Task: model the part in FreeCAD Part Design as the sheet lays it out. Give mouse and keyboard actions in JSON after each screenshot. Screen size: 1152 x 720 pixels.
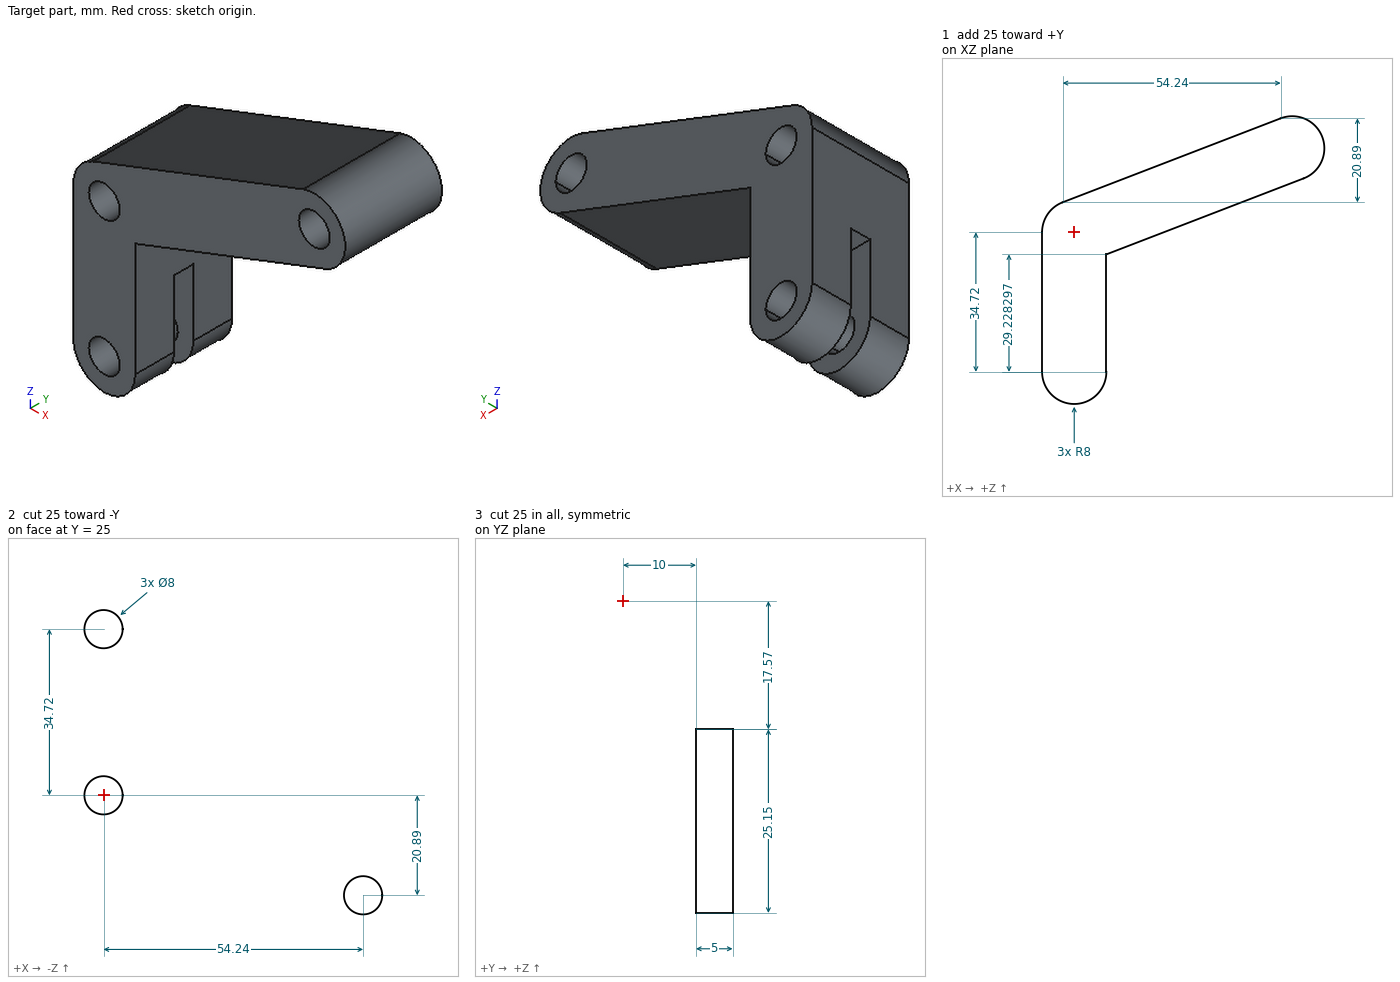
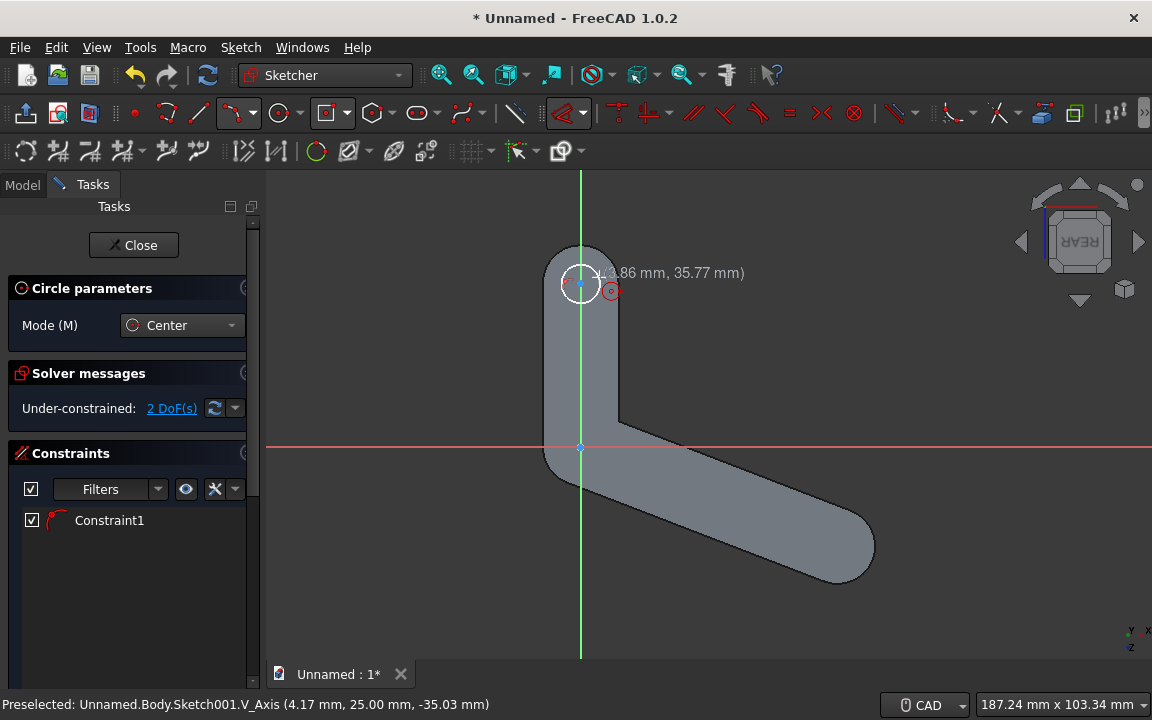
{"action": "left_click", "coordinate": [837, 546]}
{"action": "left_click", "coordinate": [851, 533]}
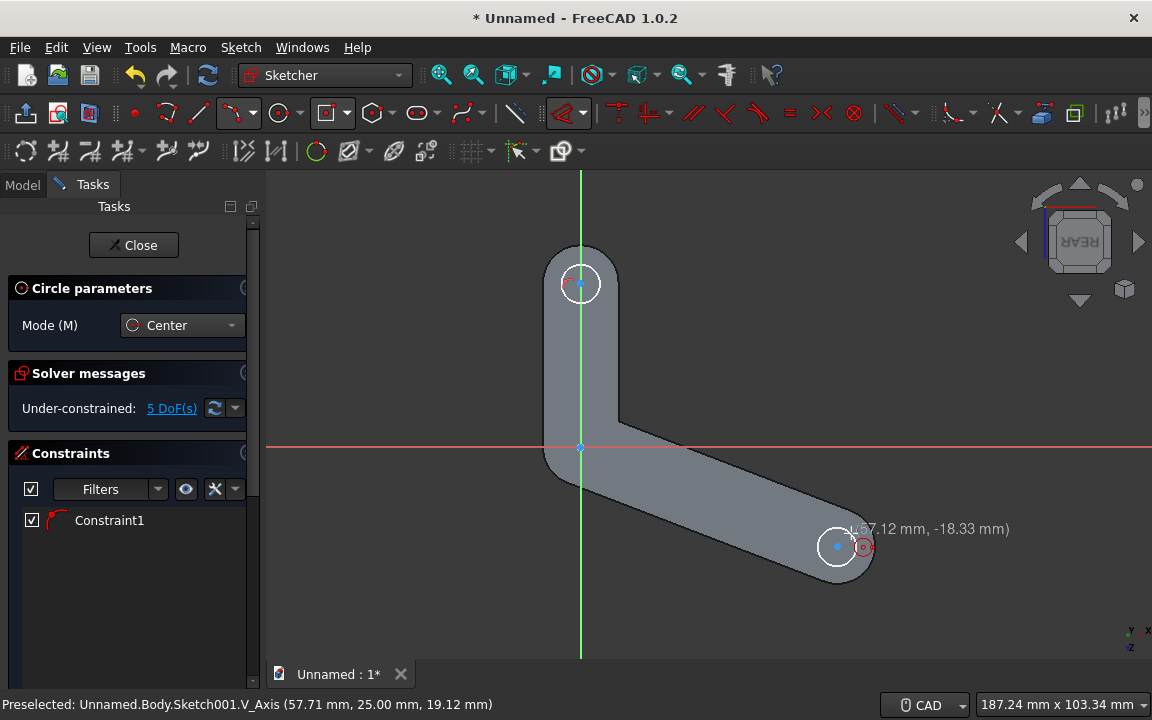
{"action": "left_click", "coordinate": [581, 447]}
{"action": "left_click", "coordinate": [594, 434]}
{"action": "key", "text": "Escape"}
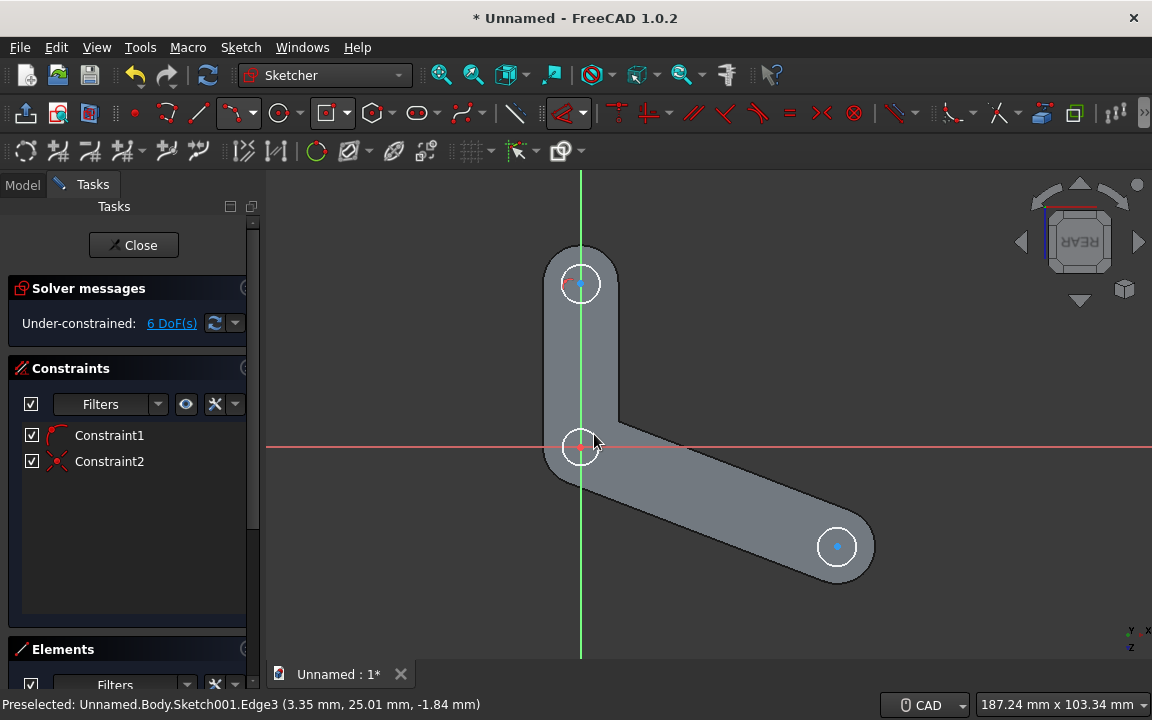
{"action": "left_click", "coordinate": [594, 270]}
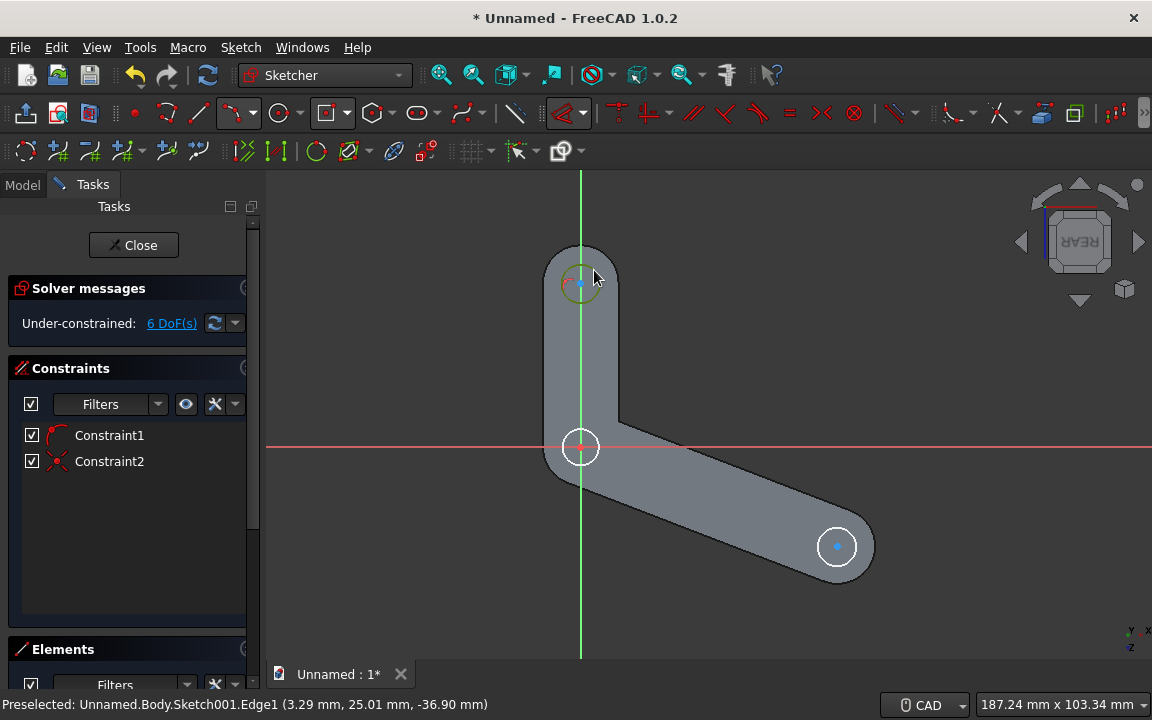
{"action": "left_click", "coordinate": [850, 533]}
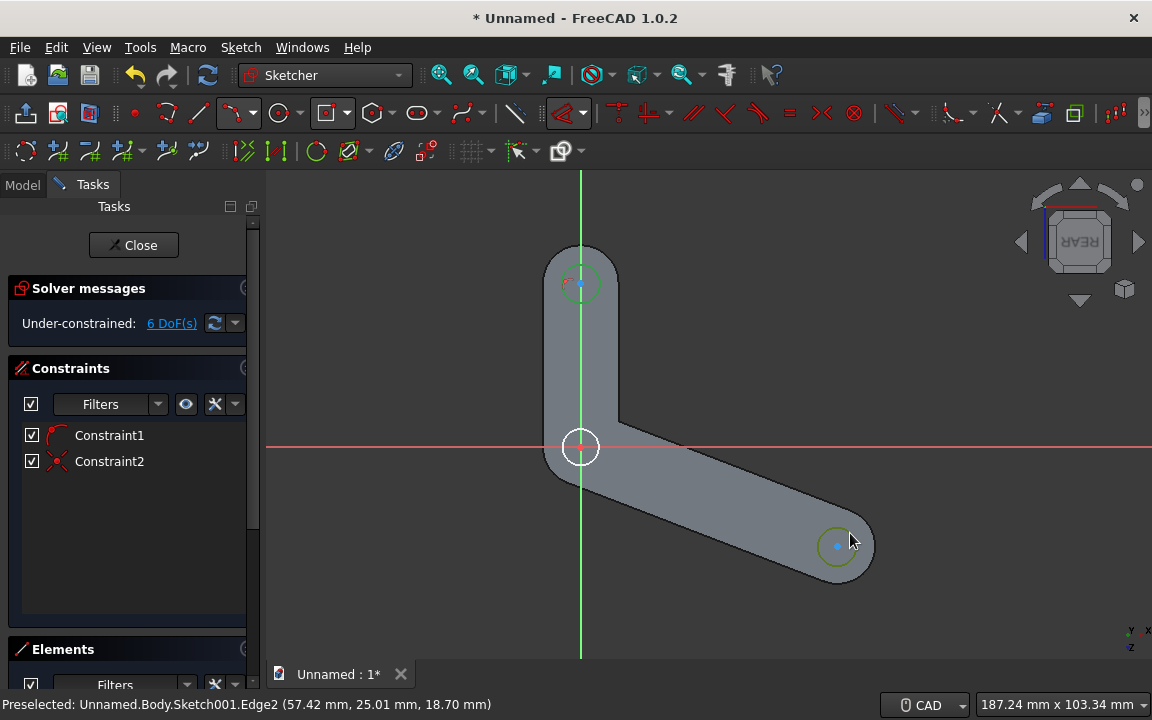
{"action": "left_click", "coordinate": [593, 434]}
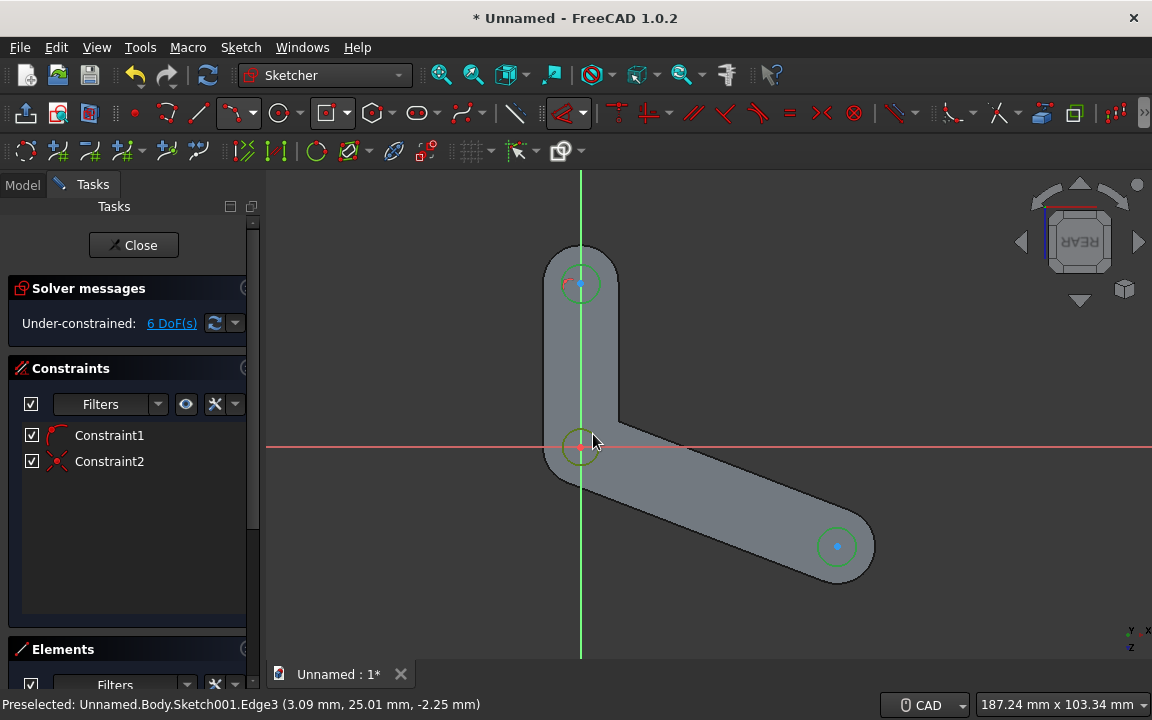
{"action": "left_click", "coordinate": [790, 114]}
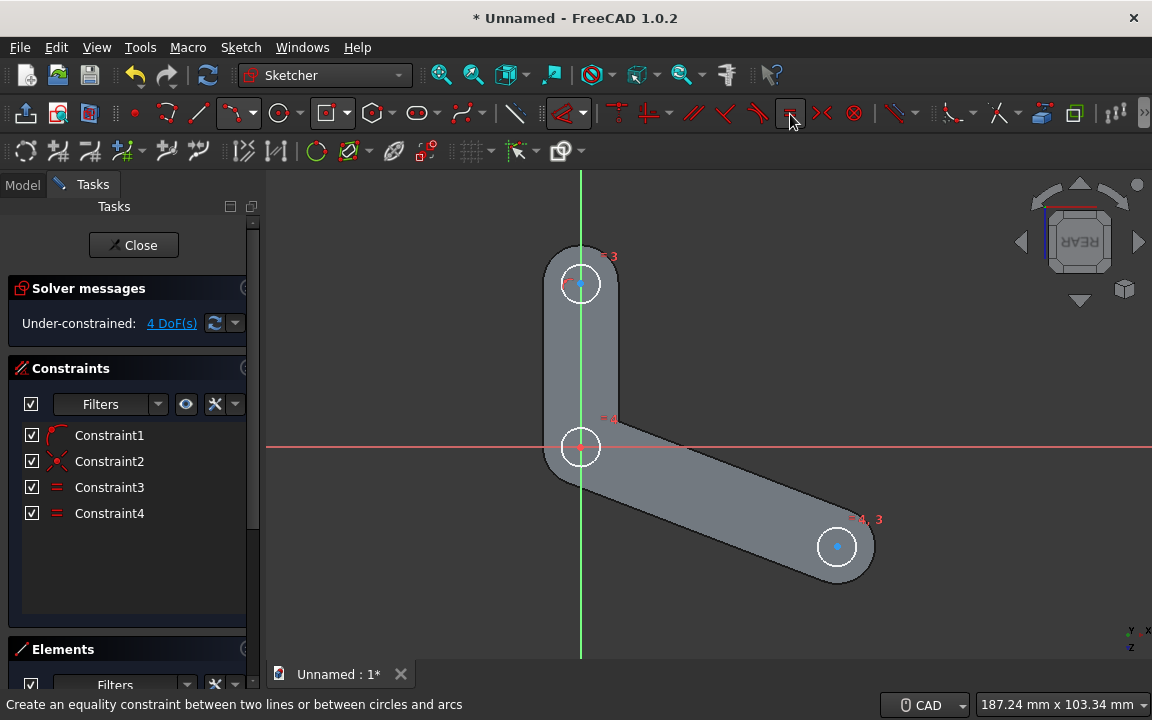
{"action": "left_click", "coordinate": [594, 270]}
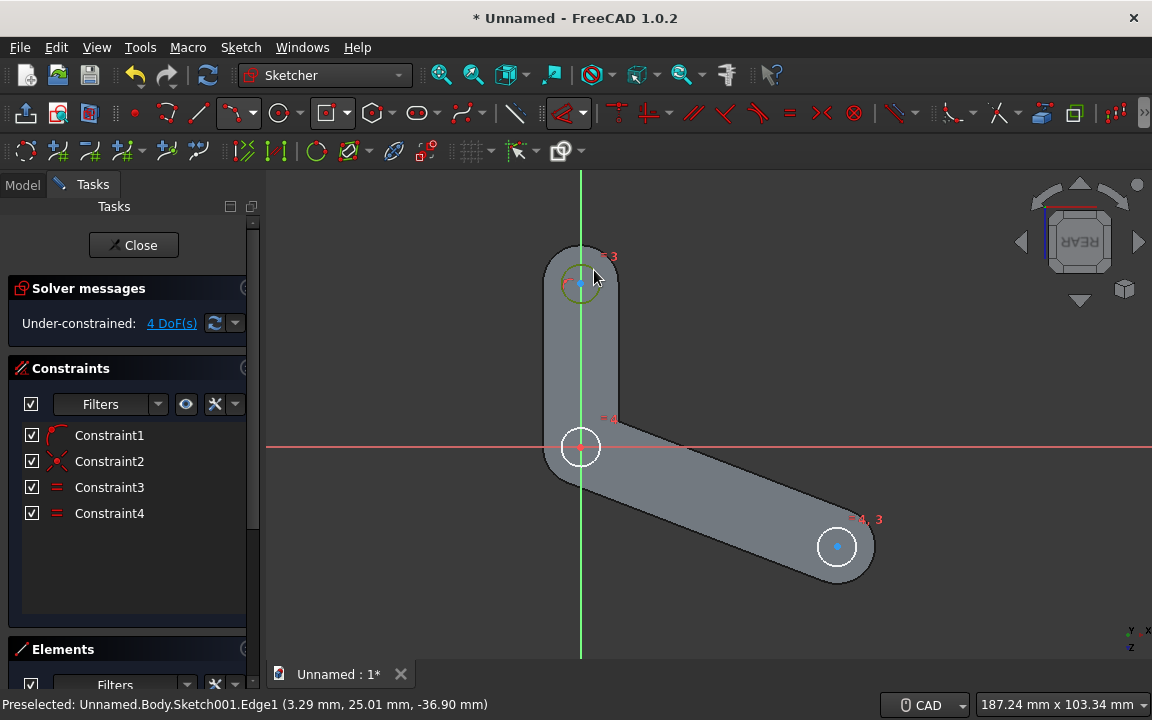
{"action": "key", "text": "k o"}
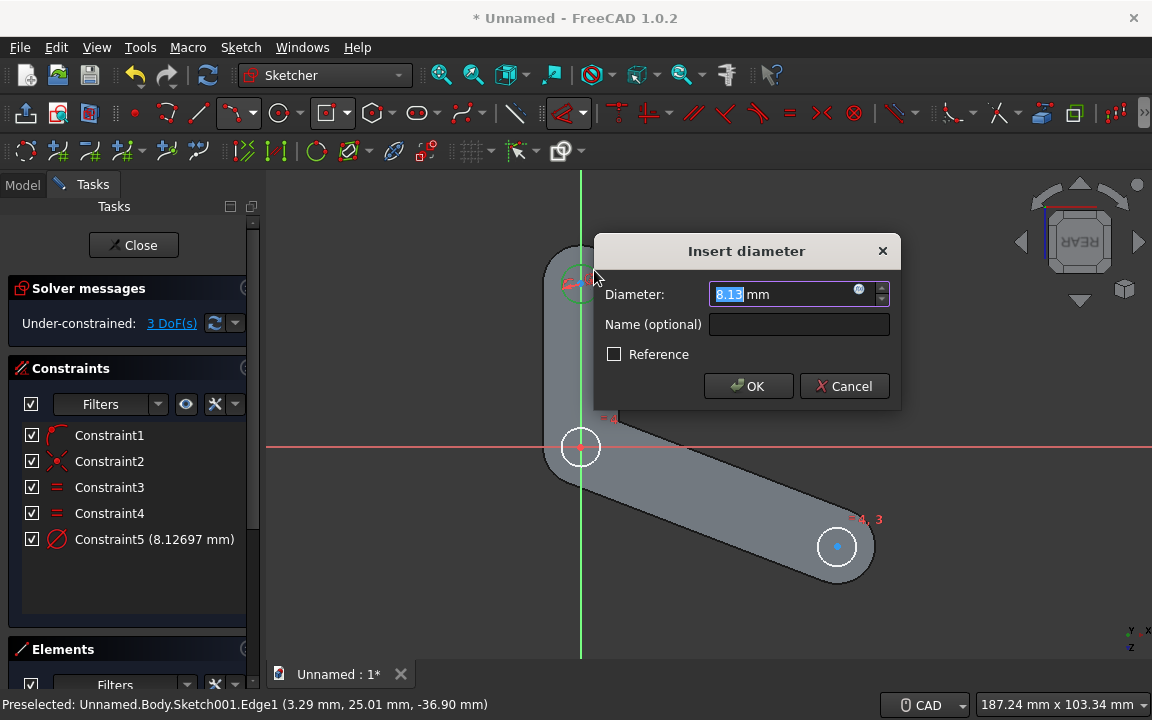
{"action": "type", "text": "8"}
{"action": "key", "text": "Return"}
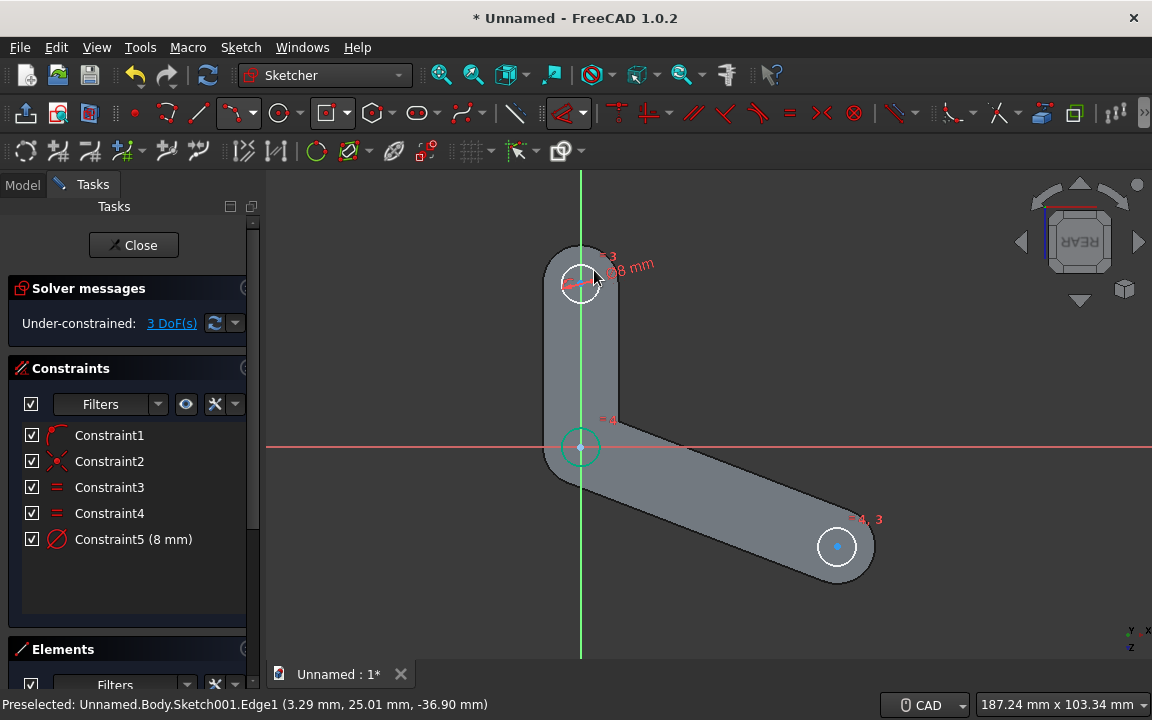
{"action": "left_click", "coordinate": [581, 284]}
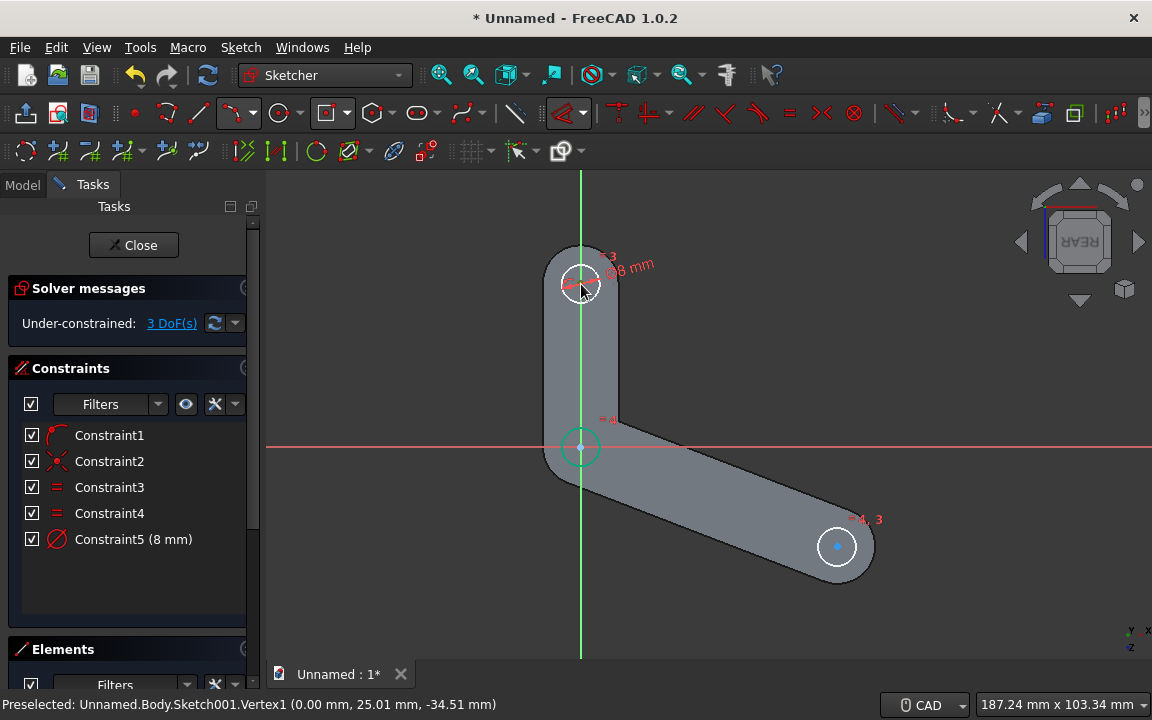
{"action": "key", "text": "i"}